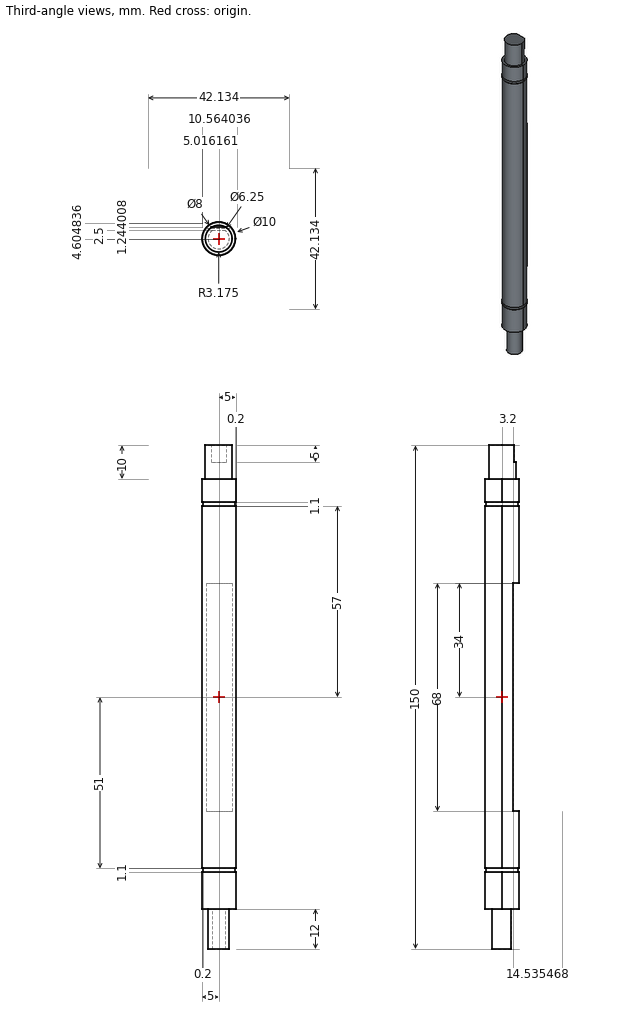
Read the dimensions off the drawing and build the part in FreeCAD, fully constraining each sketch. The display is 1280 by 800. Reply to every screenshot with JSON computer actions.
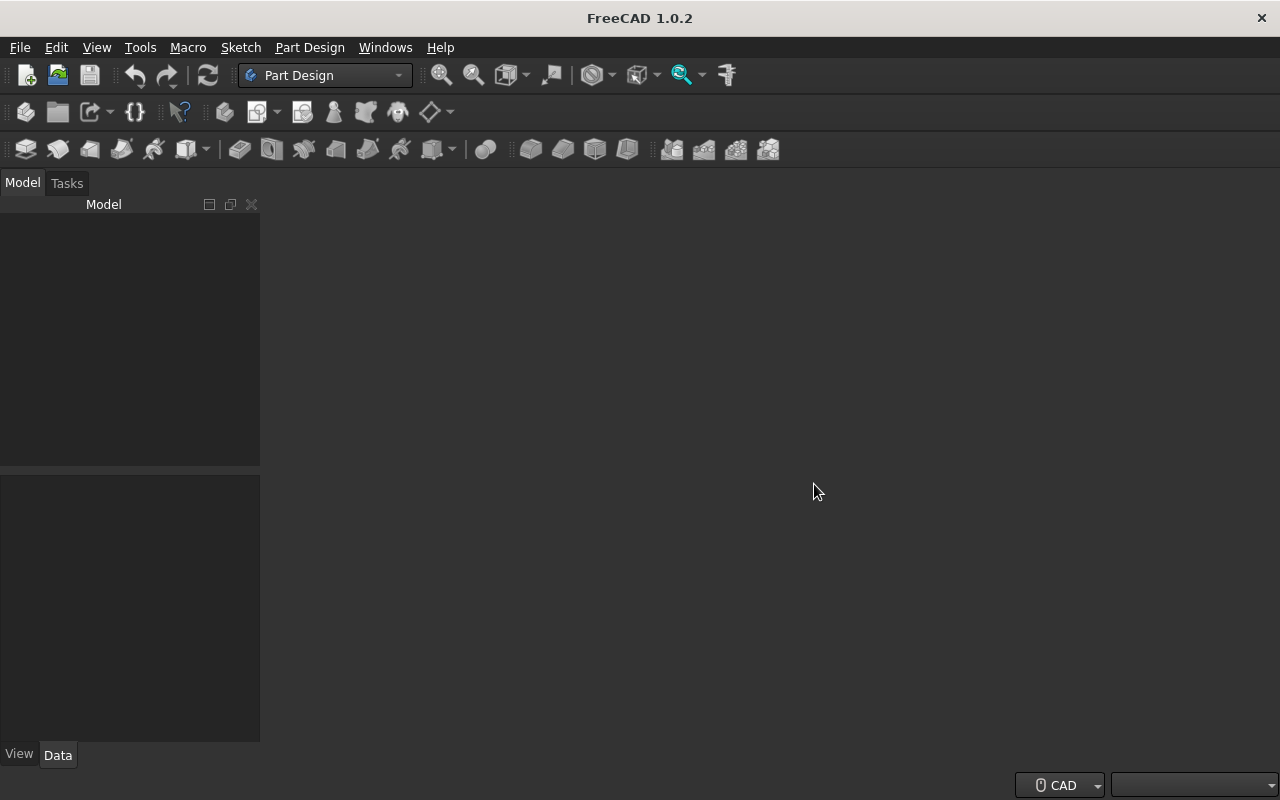
{"action": "left_click", "coordinate": [26, 76]}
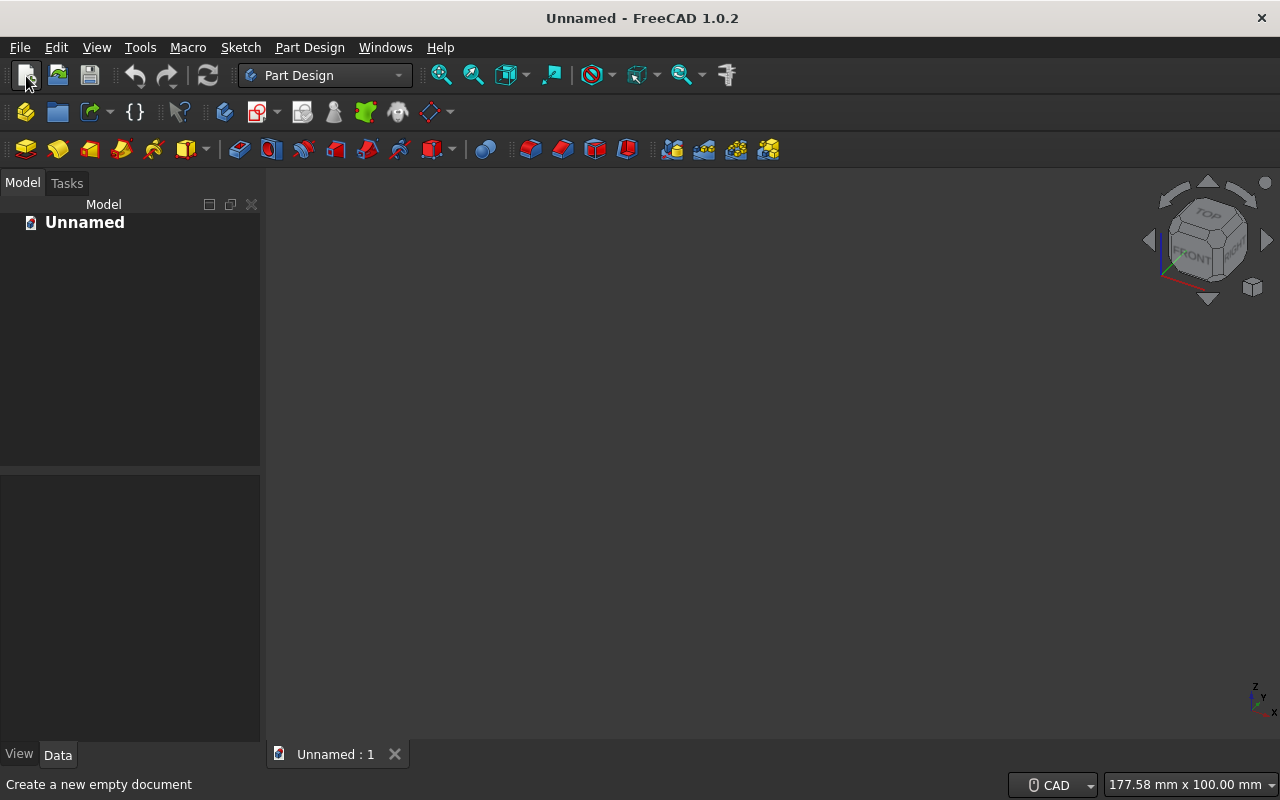
{"action": "left_click", "coordinate": [258, 112]}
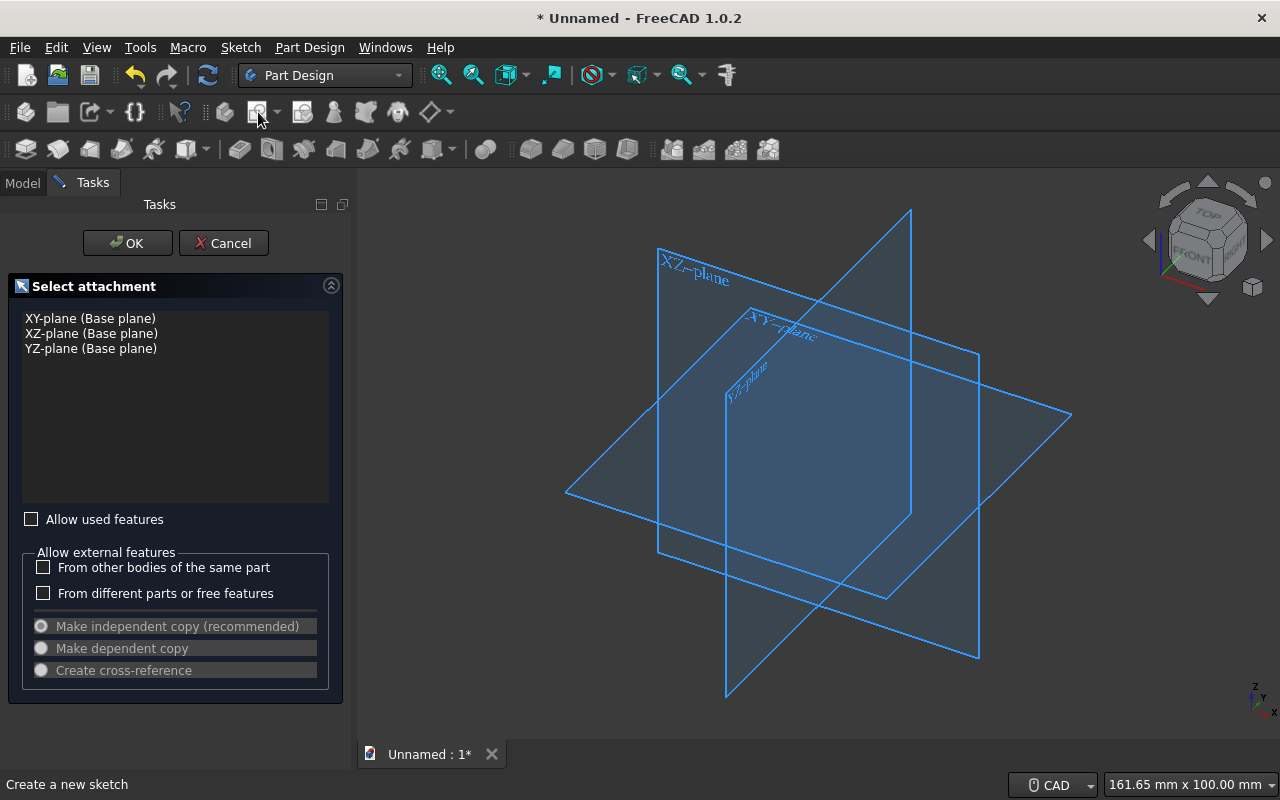
{"action": "left_click", "coordinate": [82, 318]}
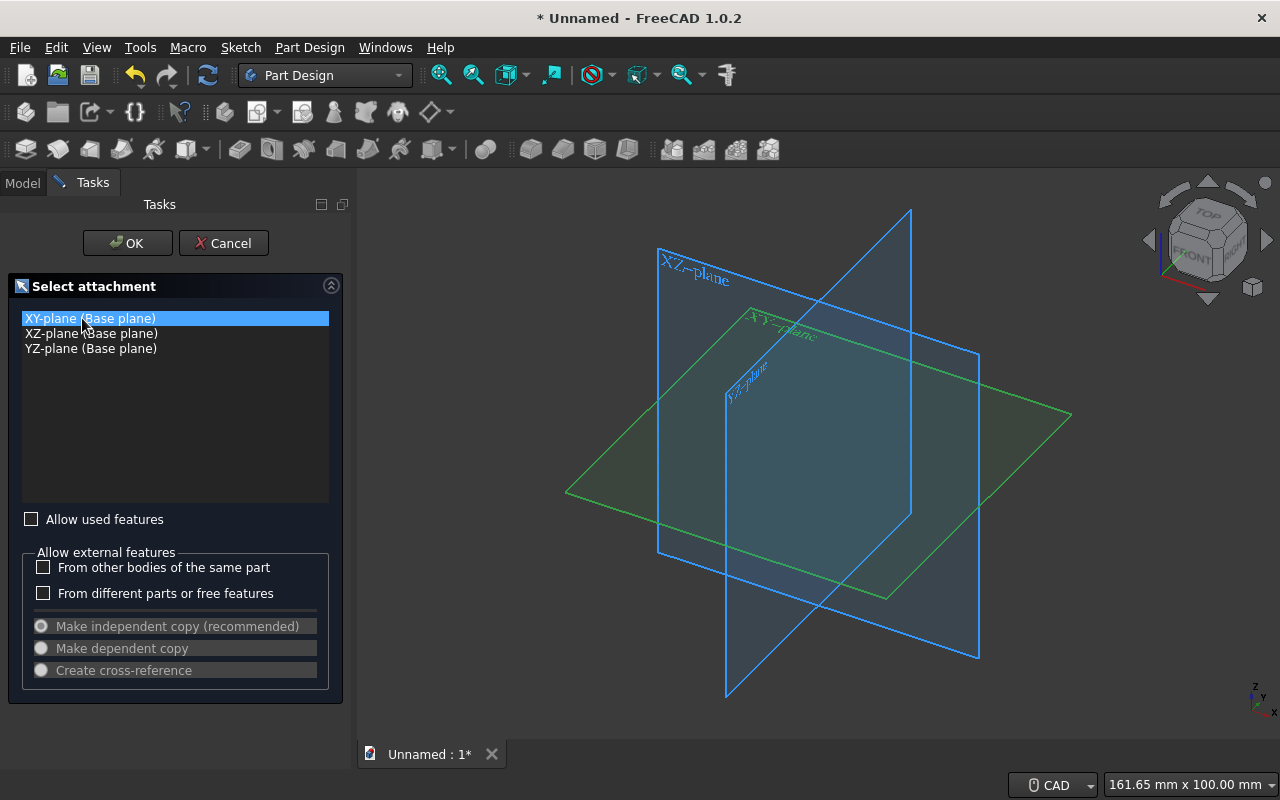
{"action": "left_click", "coordinate": [128, 243]}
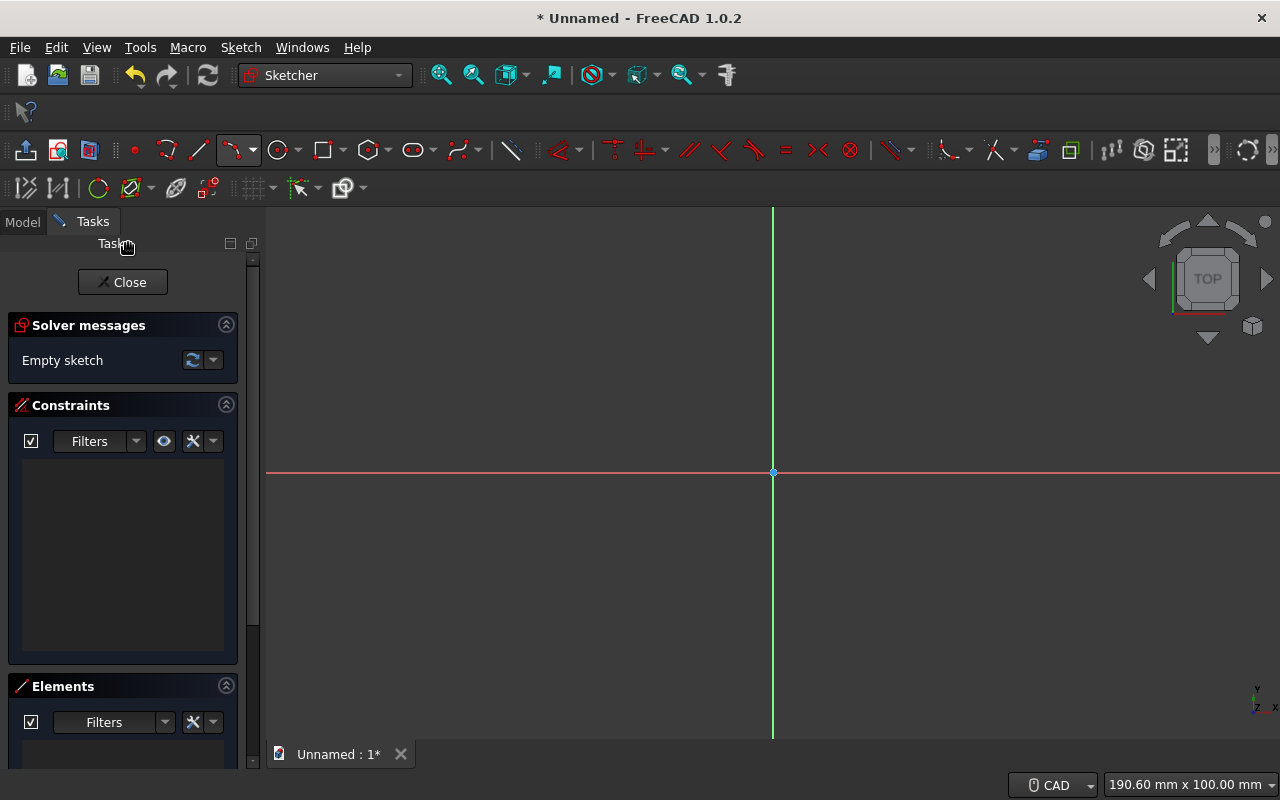
{"action": "scroll", "coordinate": [787, 473], "scroll_direction": "up", "scroll_amount": 9}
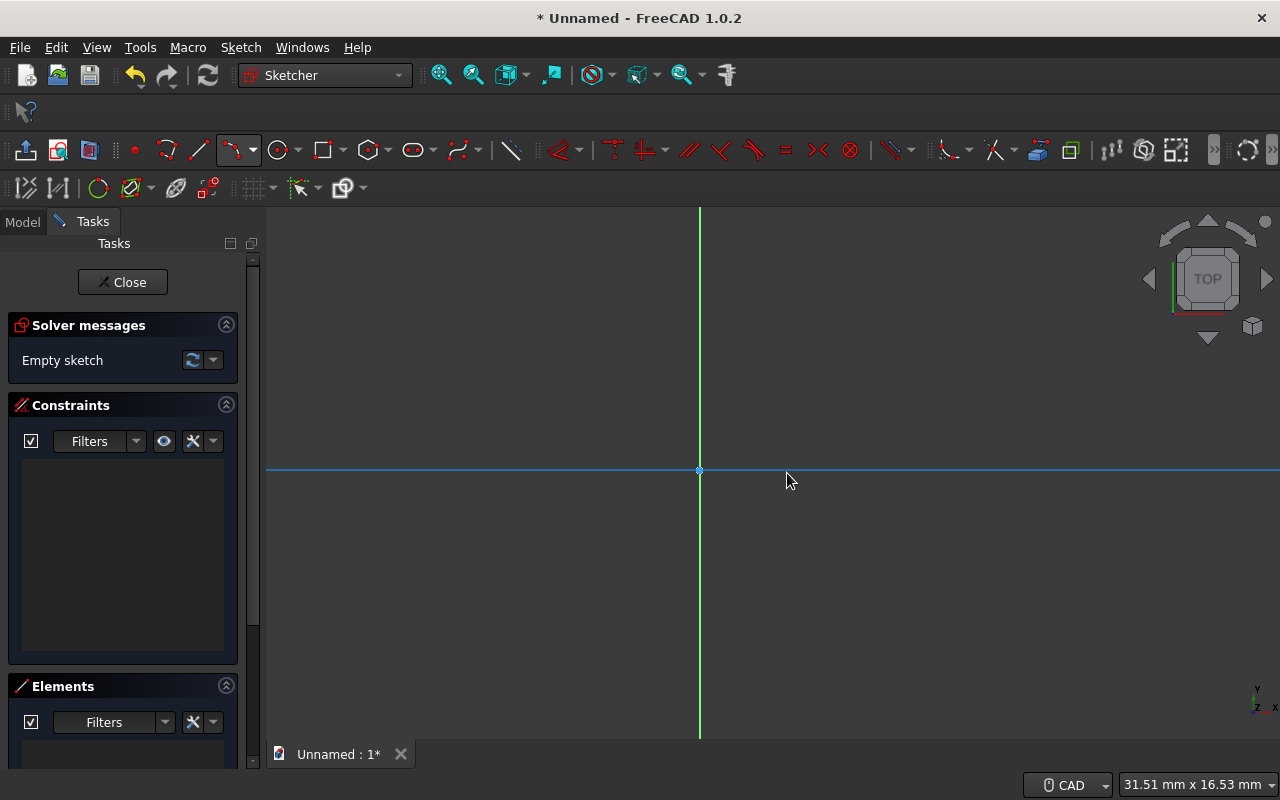
{"action": "left_click", "coordinate": [278, 150]}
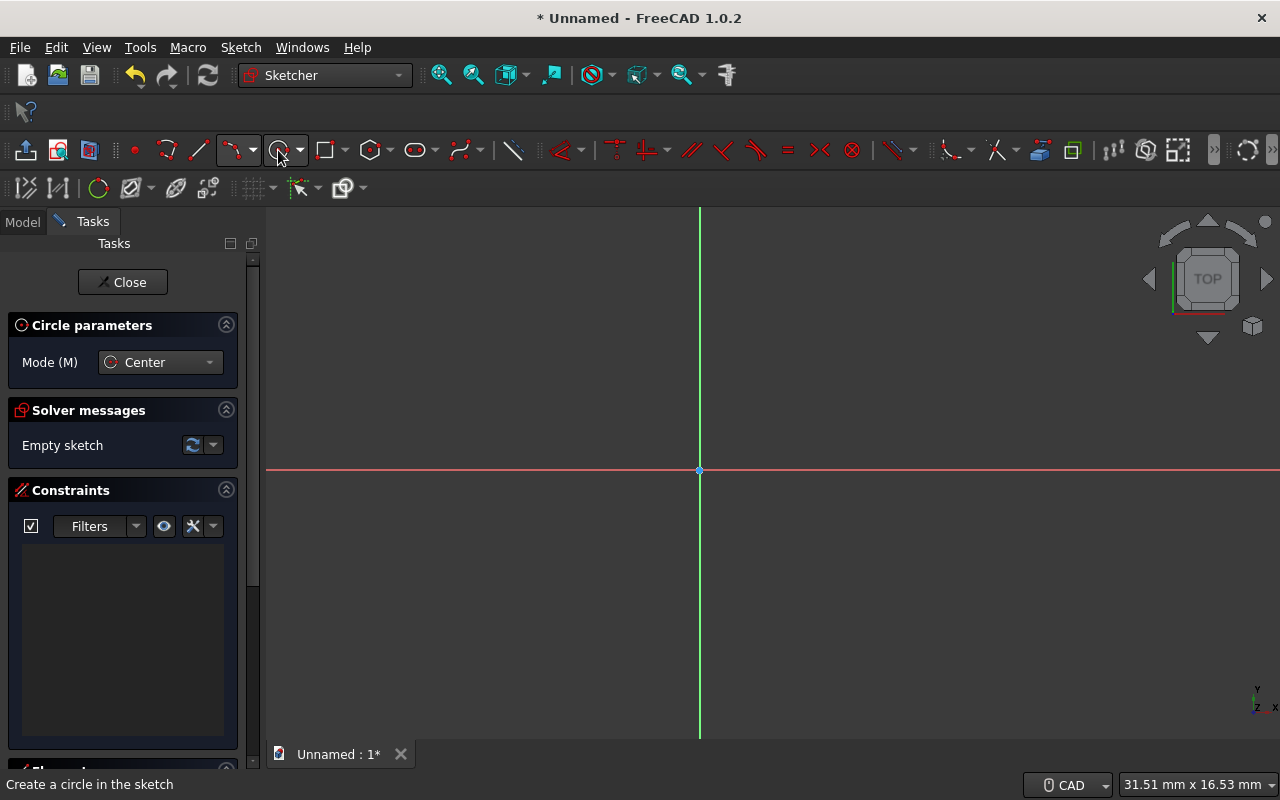
{"action": "left_click", "coordinate": [700, 470]}
{"action": "left_click", "coordinate": [813, 357]}
{"action": "key", "text": "Escape"}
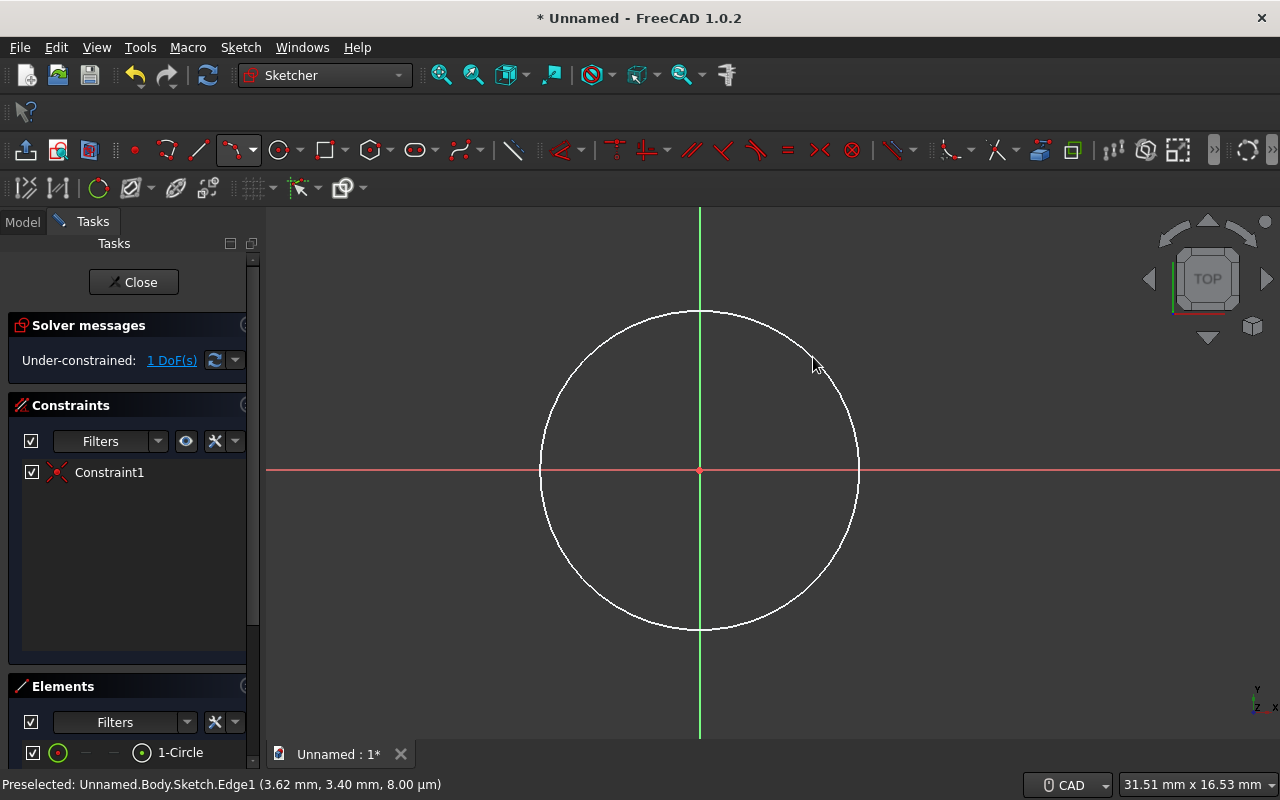
{"action": "left_click", "coordinate": [812, 357]}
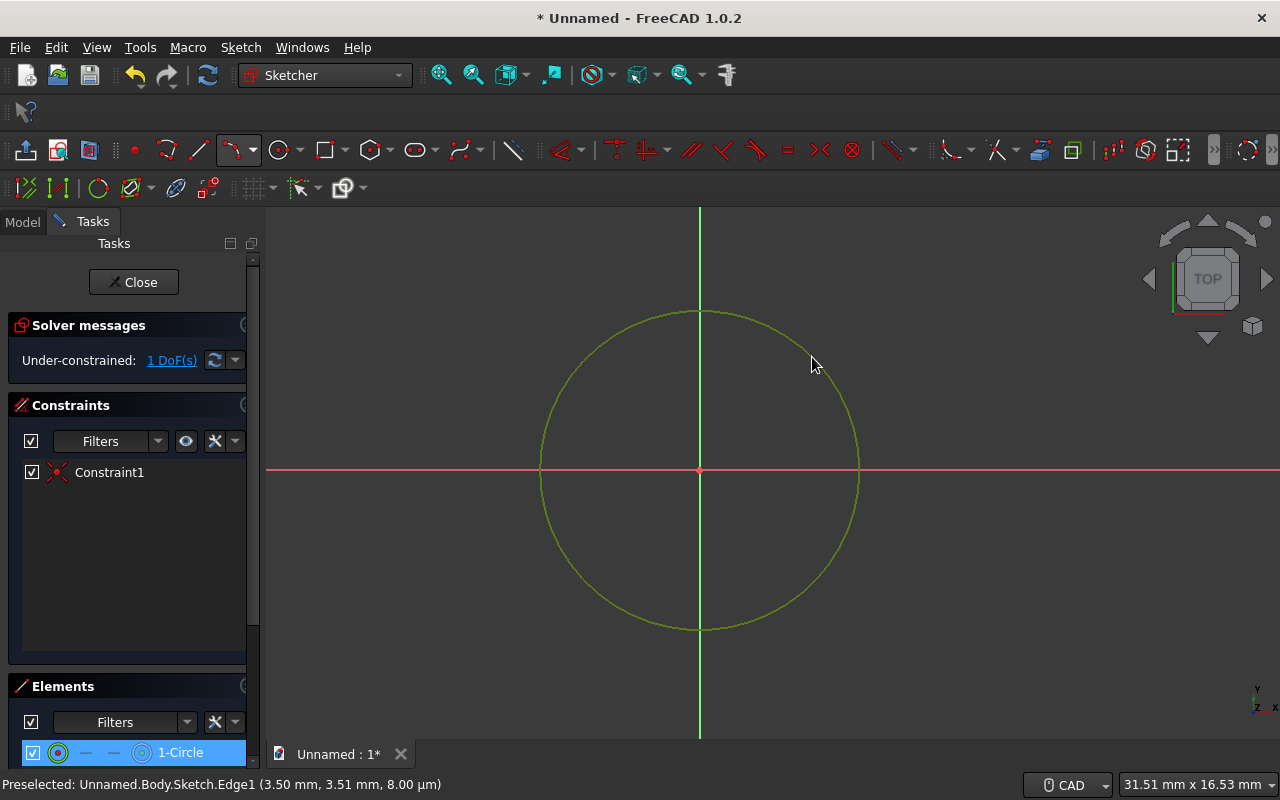
{"action": "key", "text": "k o"}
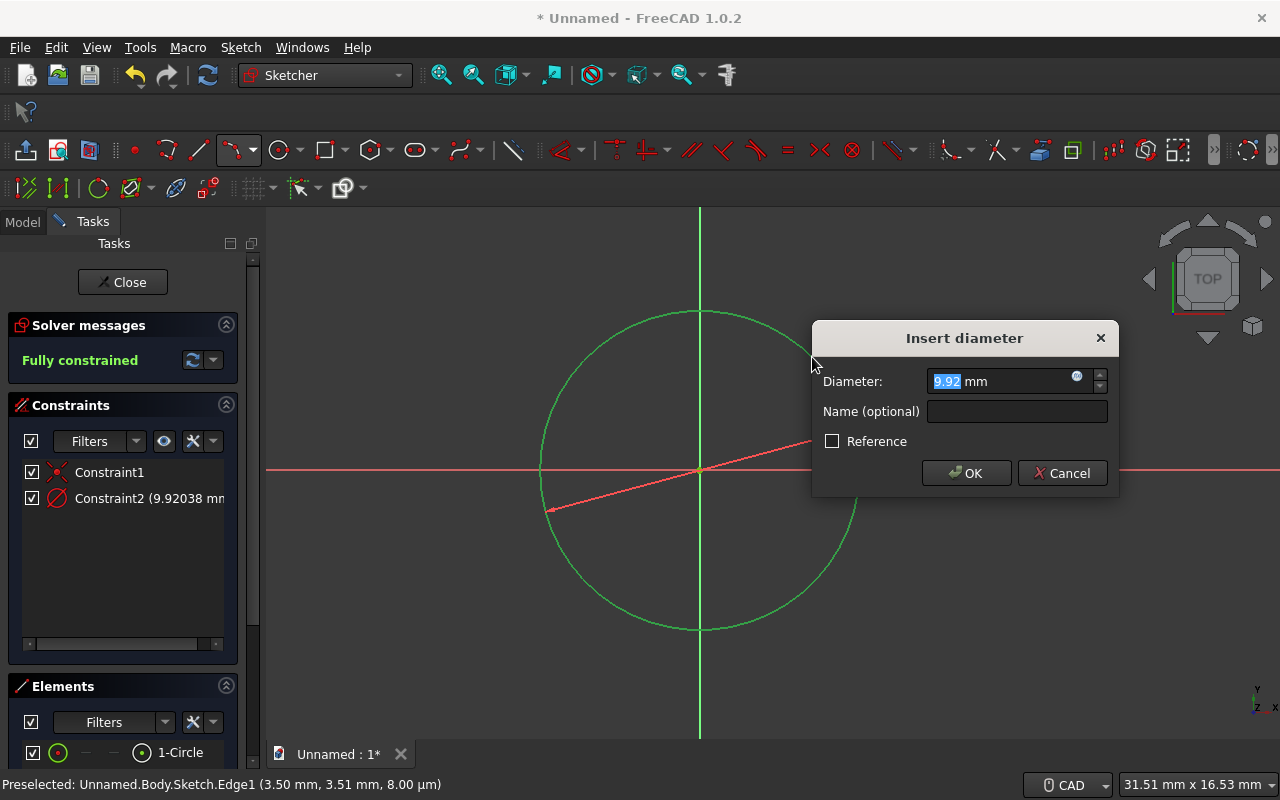
{"action": "type", "text": "10"}
{"action": "key", "text": "Return"}